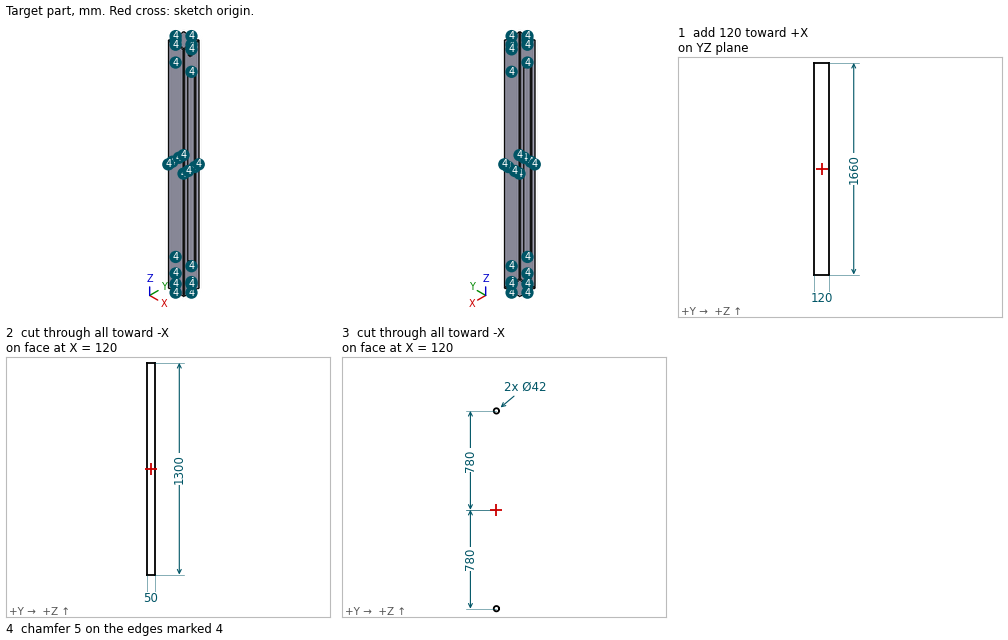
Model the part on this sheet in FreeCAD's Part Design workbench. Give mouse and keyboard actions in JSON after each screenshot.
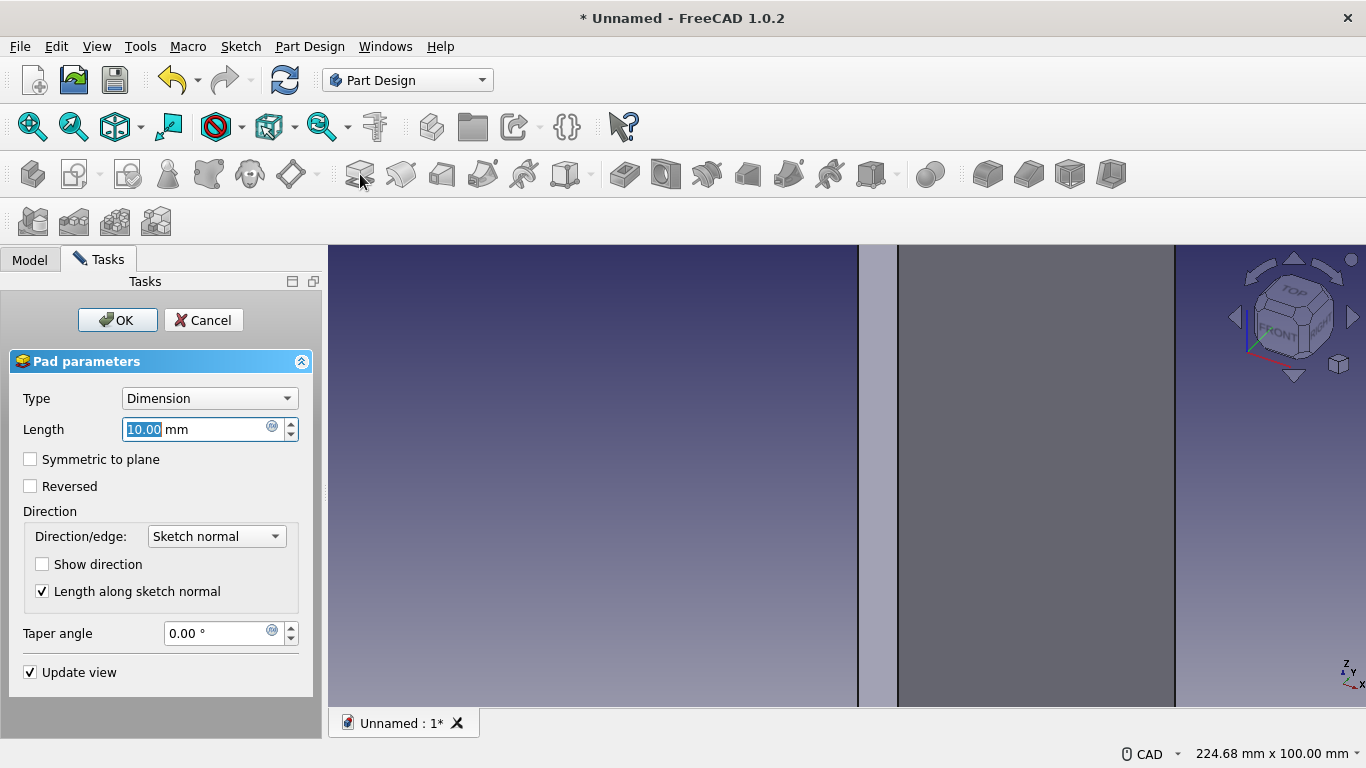
{"action": "type", "text": "120"}
{"action": "key", "text": "Tab"}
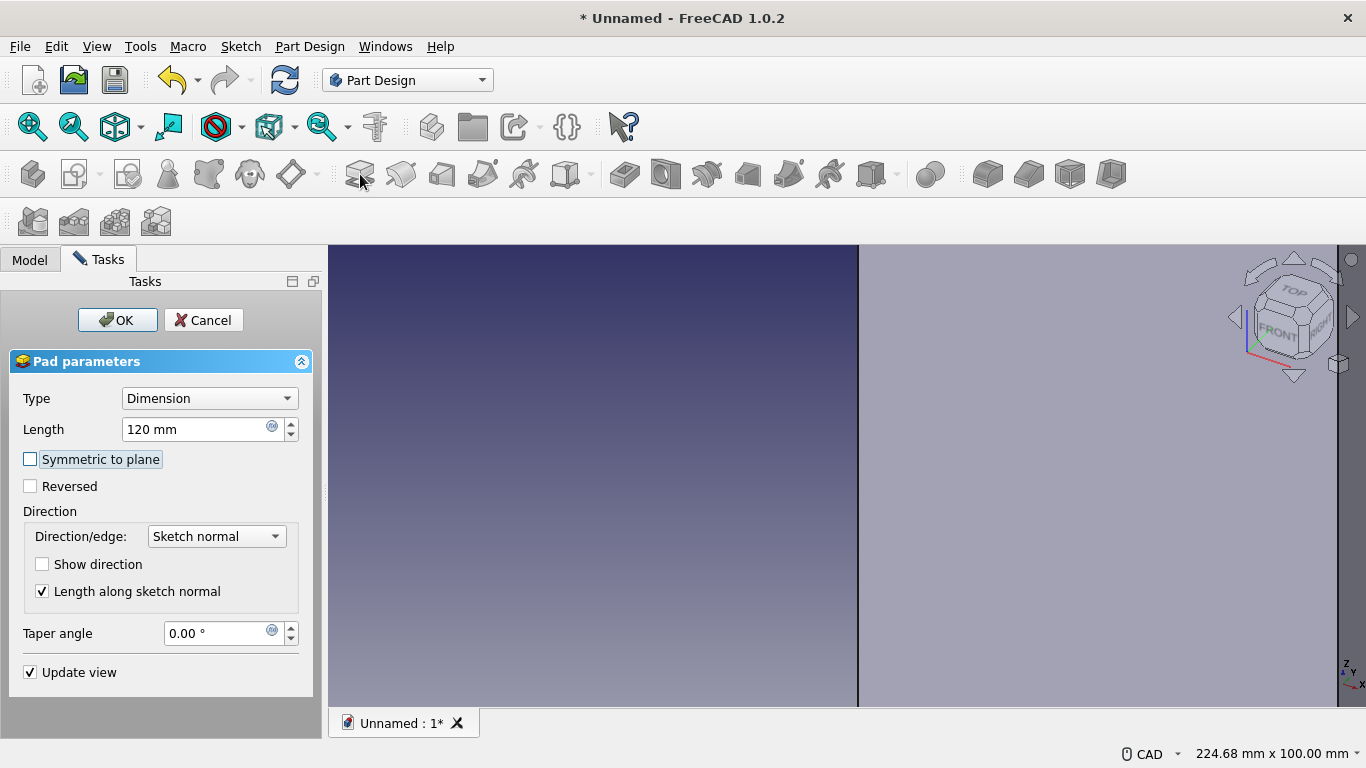
{"action": "left_click", "coordinate": [118, 320]}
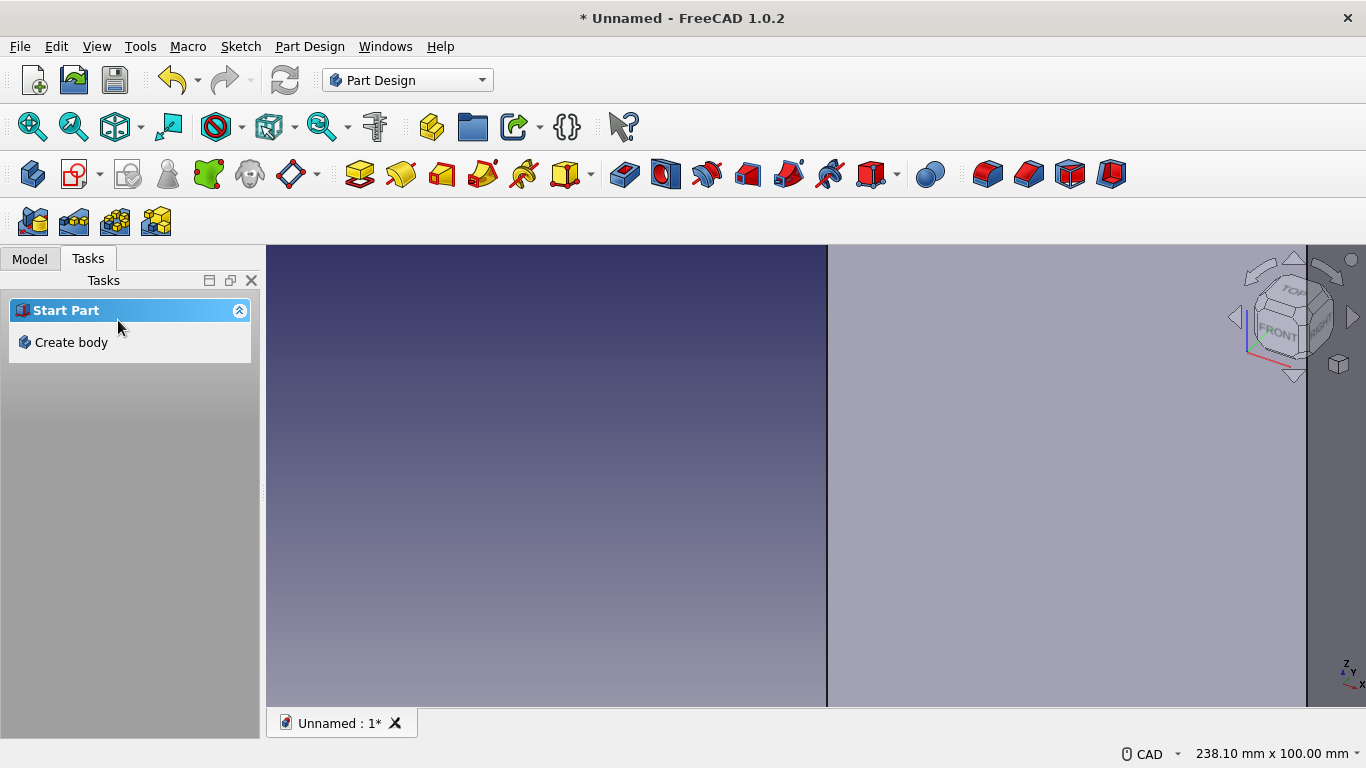
{"action": "left_click", "coordinate": [33, 128]}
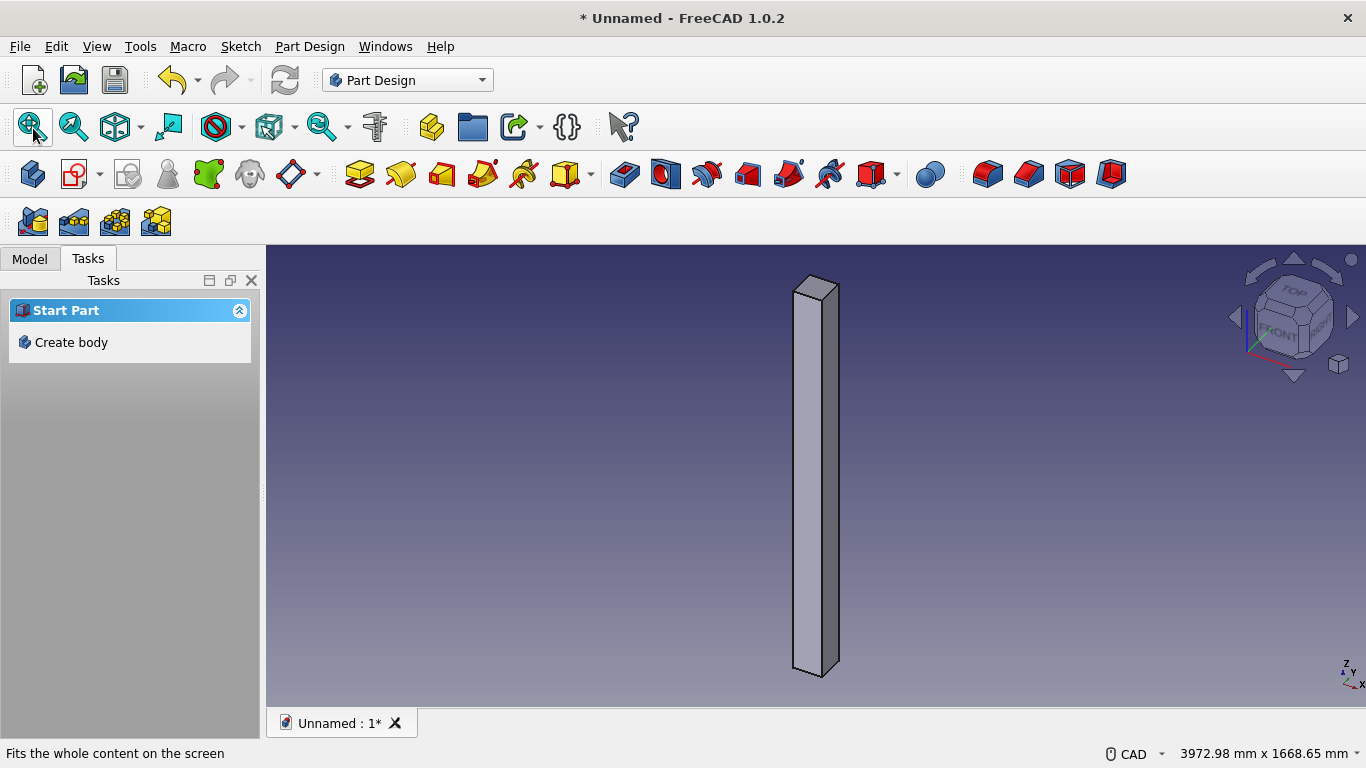
{"action": "key", "text": "0"}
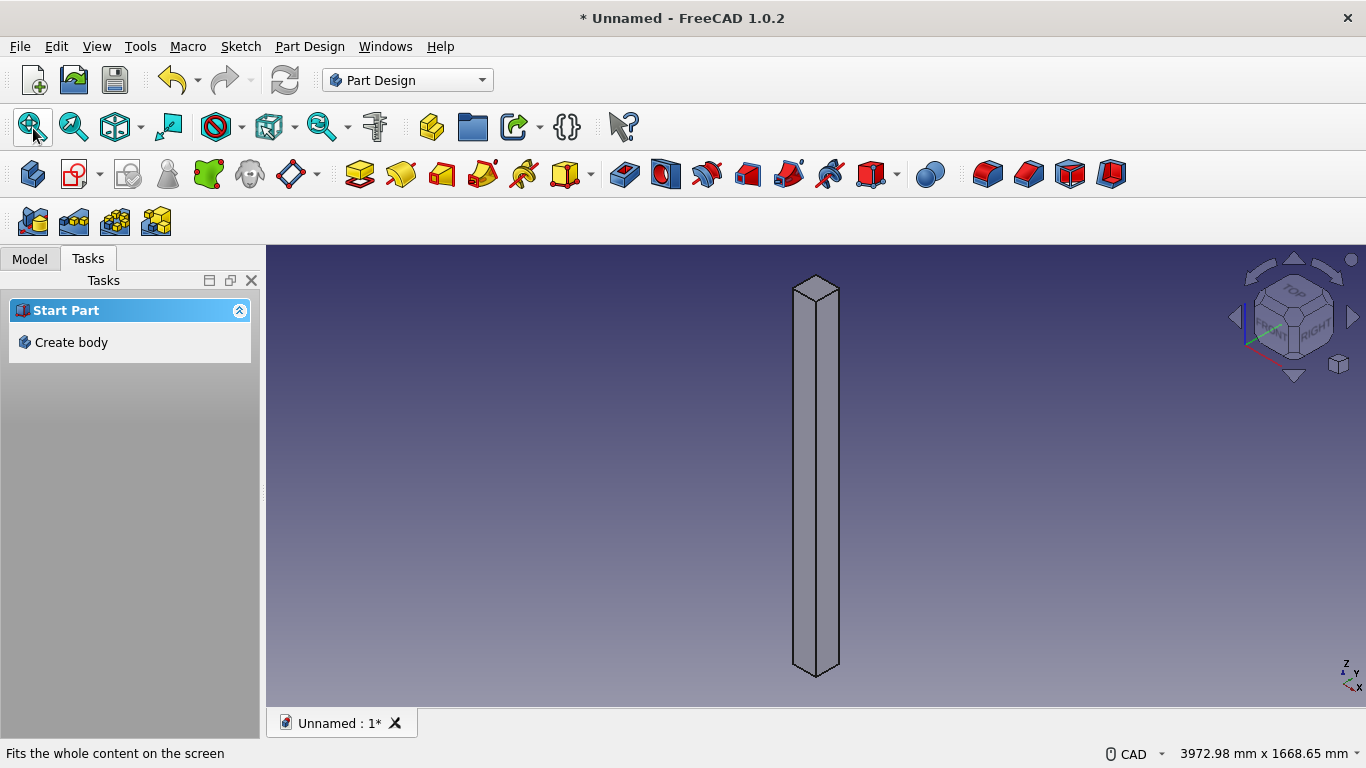
{"action": "left_click", "coordinate": [828, 643]}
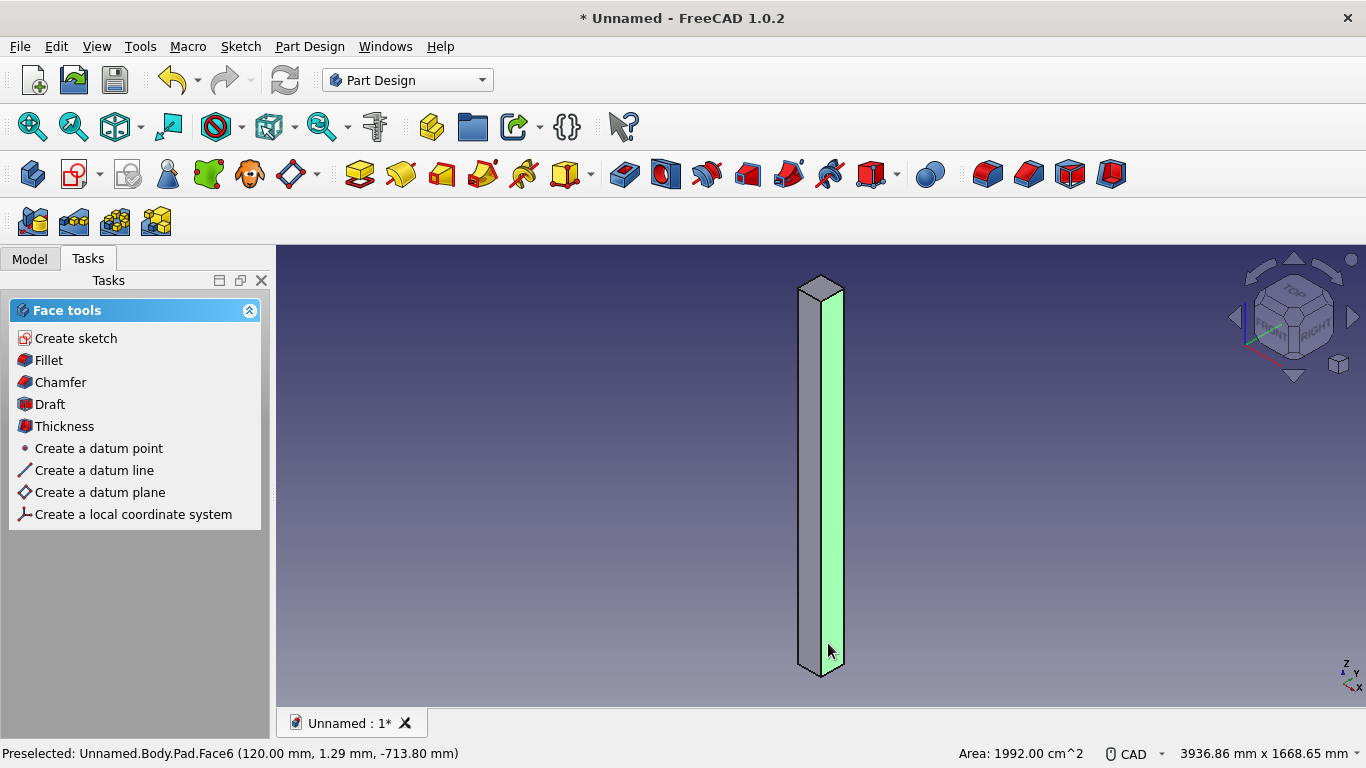
{"action": "left_click", "coordinate": [74, 174]}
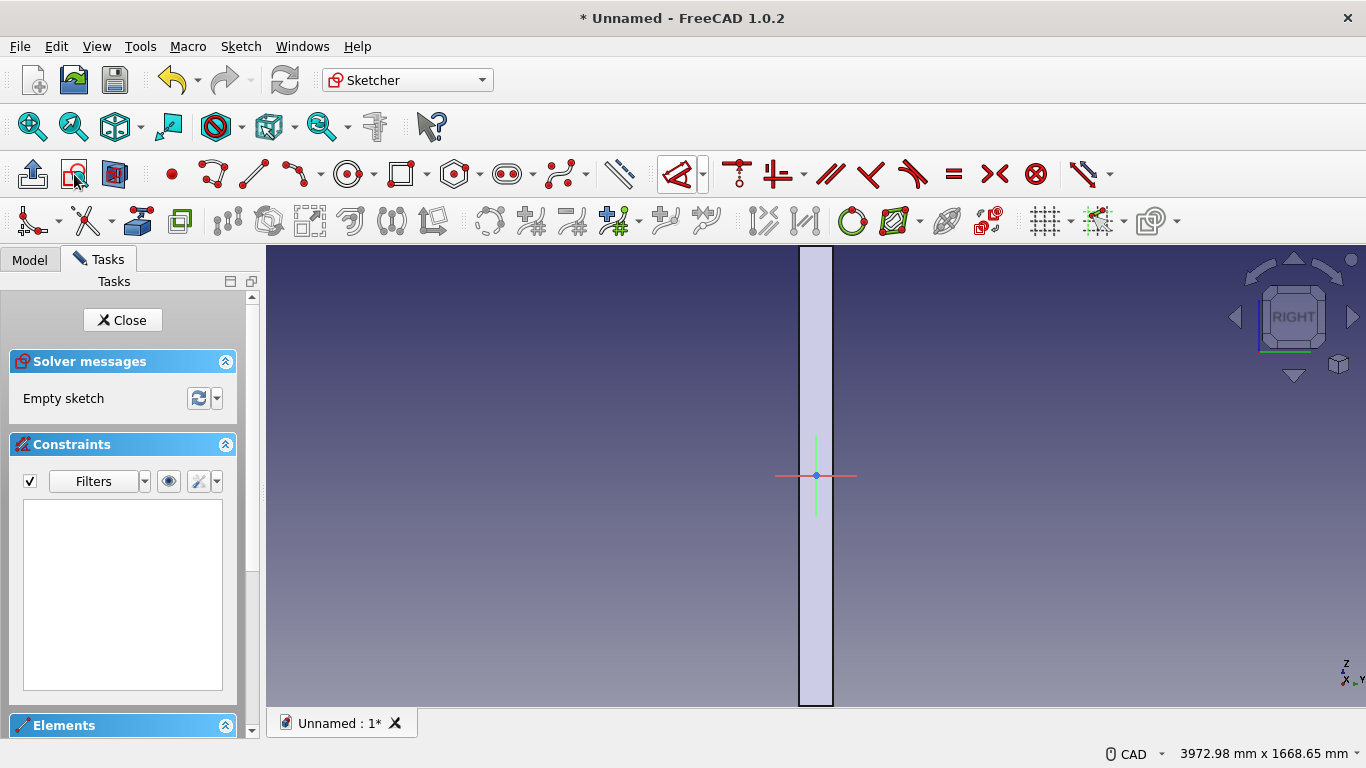
{"action": "scroll", "coordinate": [438, 476], "scroll_direction": "down", "scroll_amount": 1}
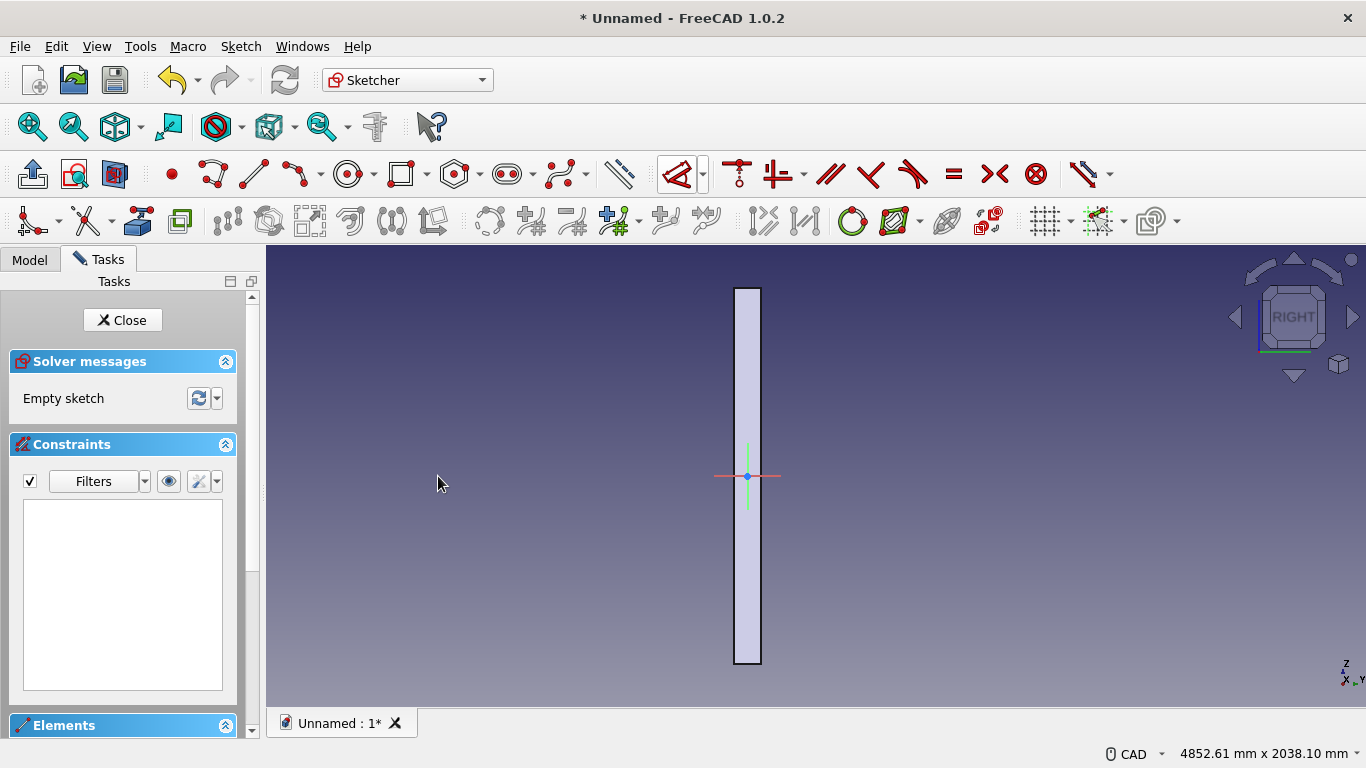
{"action": "key", "text": "g v"}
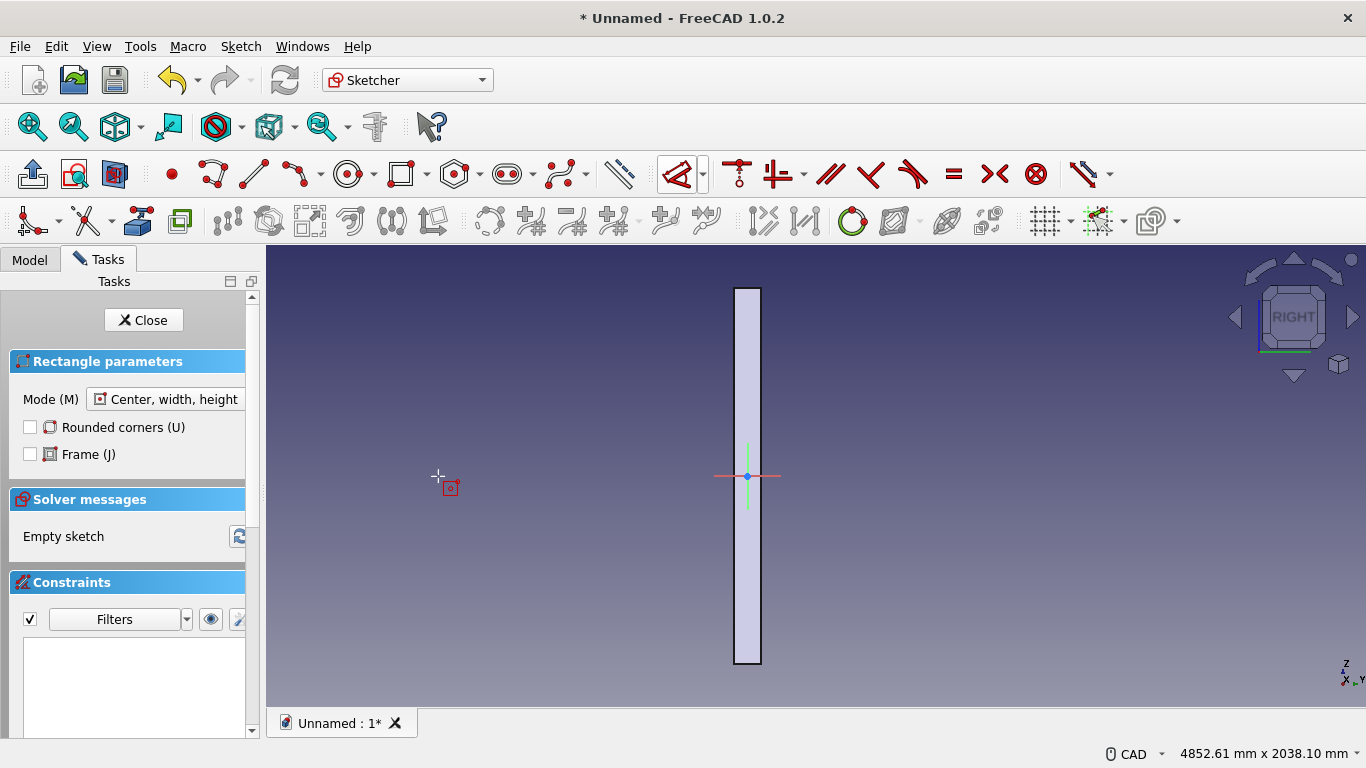
{"action": "scroll", "coordinate": [748, 476], "scroll_direction": "up", "scroll_amount": 6}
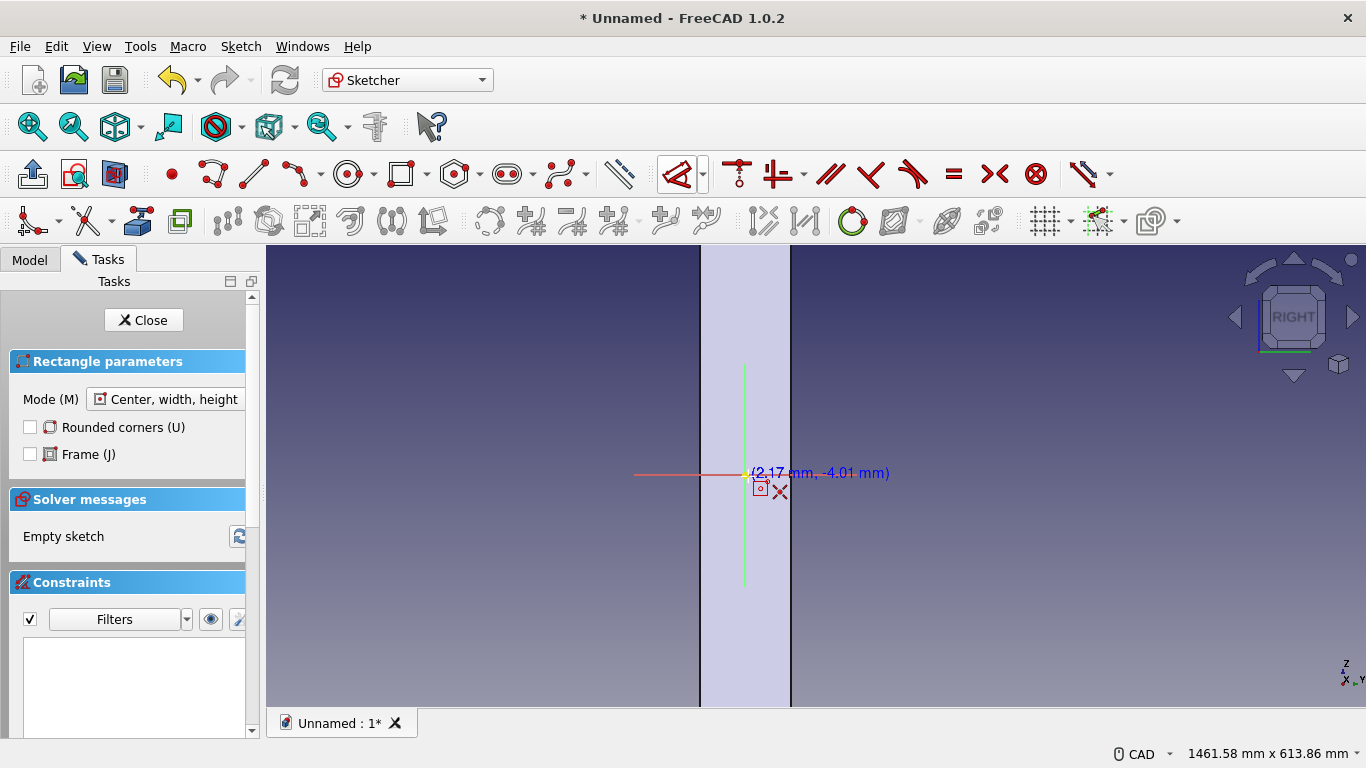
{"action": "left_click", "coordinate": [745, 475]}